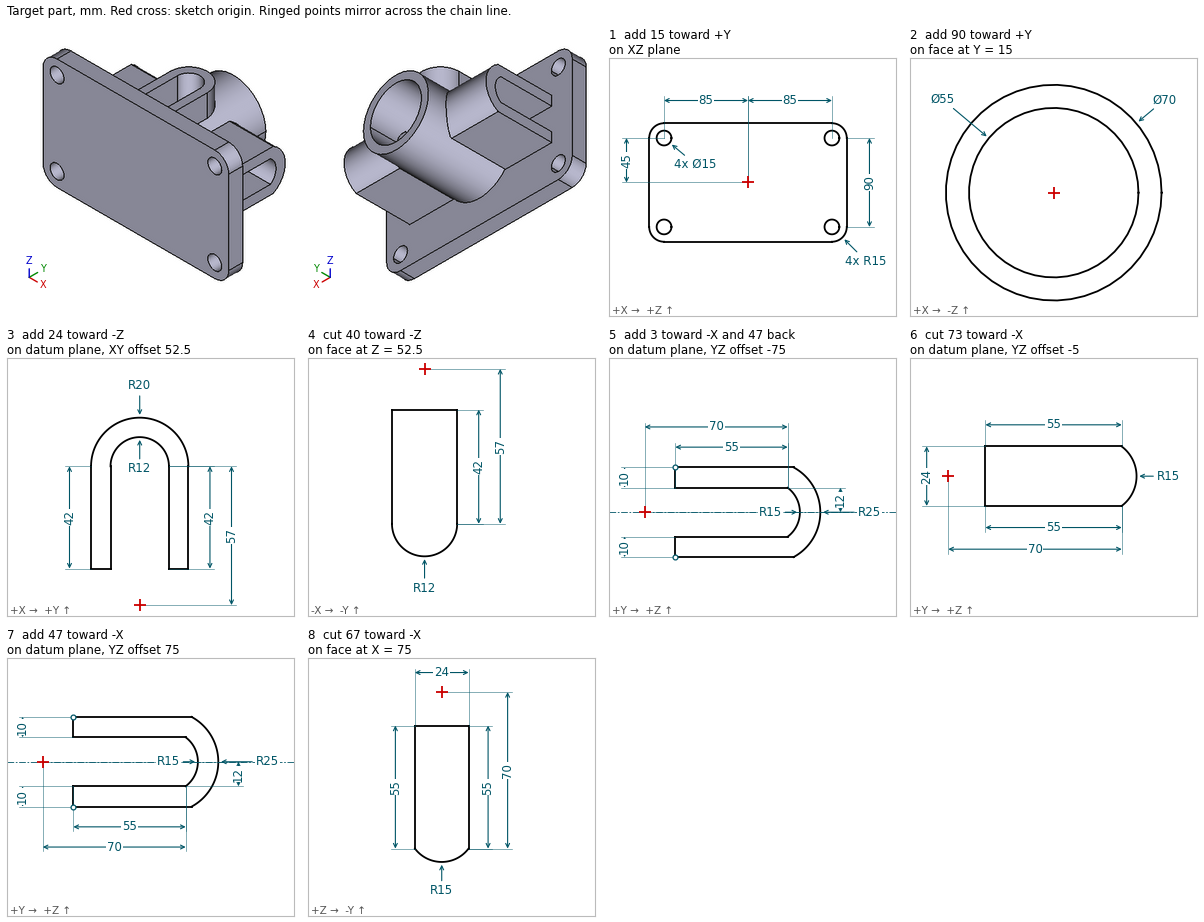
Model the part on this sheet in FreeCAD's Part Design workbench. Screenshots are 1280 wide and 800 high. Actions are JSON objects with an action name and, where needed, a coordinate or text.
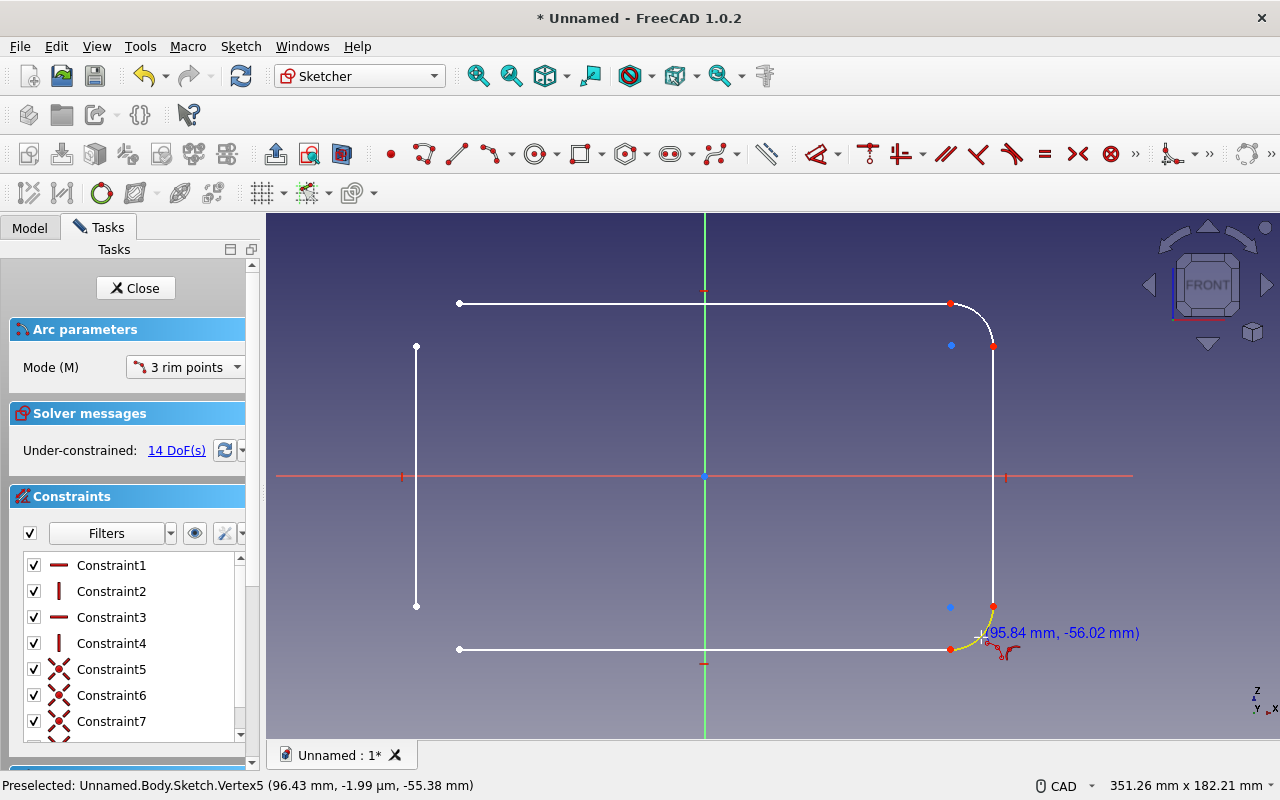
{"action": "left_click", "coordinate": [459, 650]}
{"action": "left_click", "coordinate": [416, 607]}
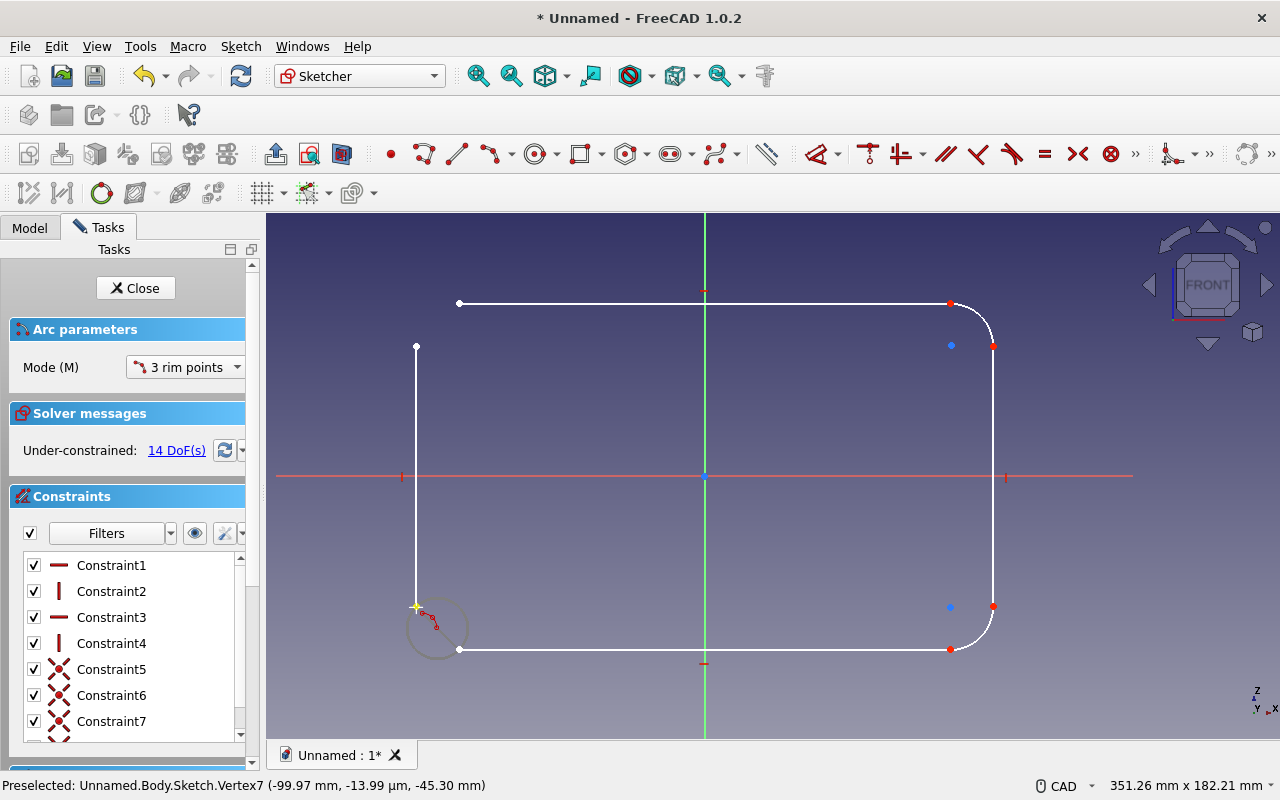
{"action": "scroll", "coordinate": [429, 637], "scroll_direction": "up", "scroll_amount": 2}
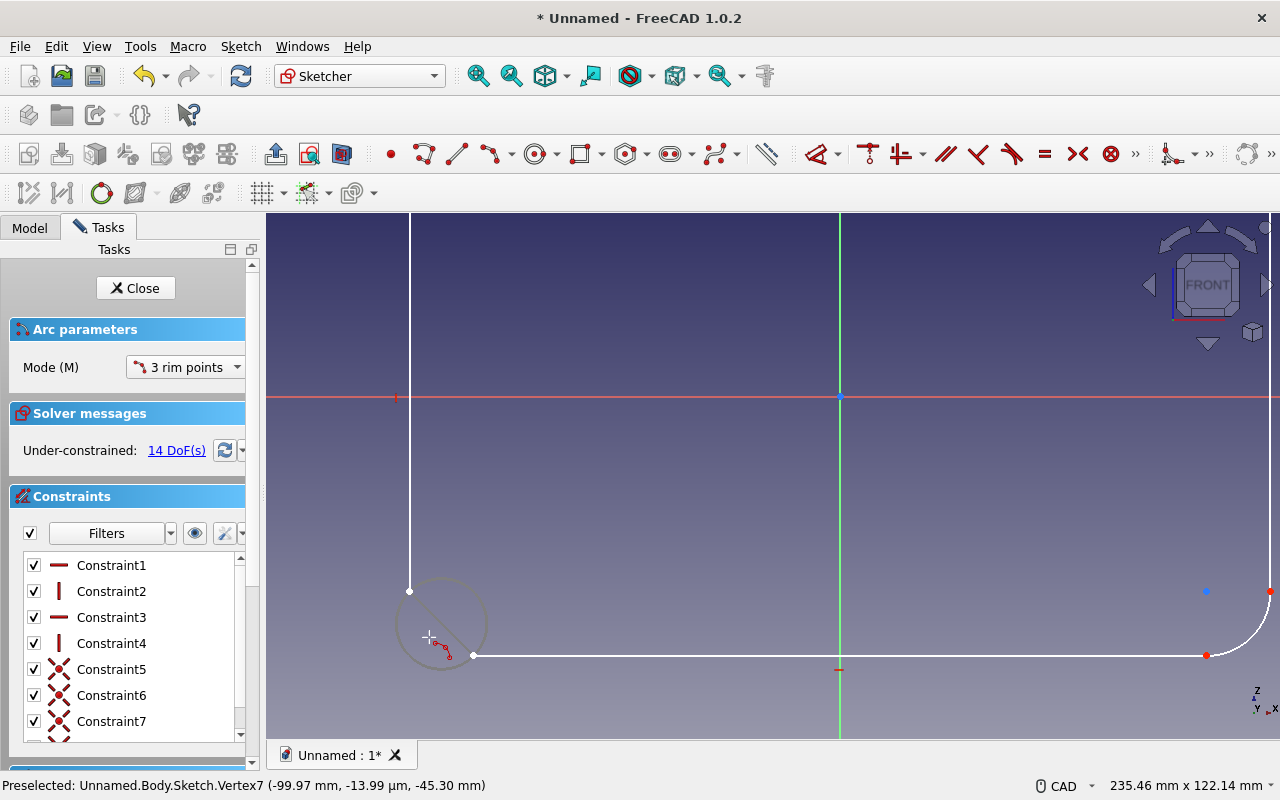
{"action": "left_click", "coordinate": [428, 636]}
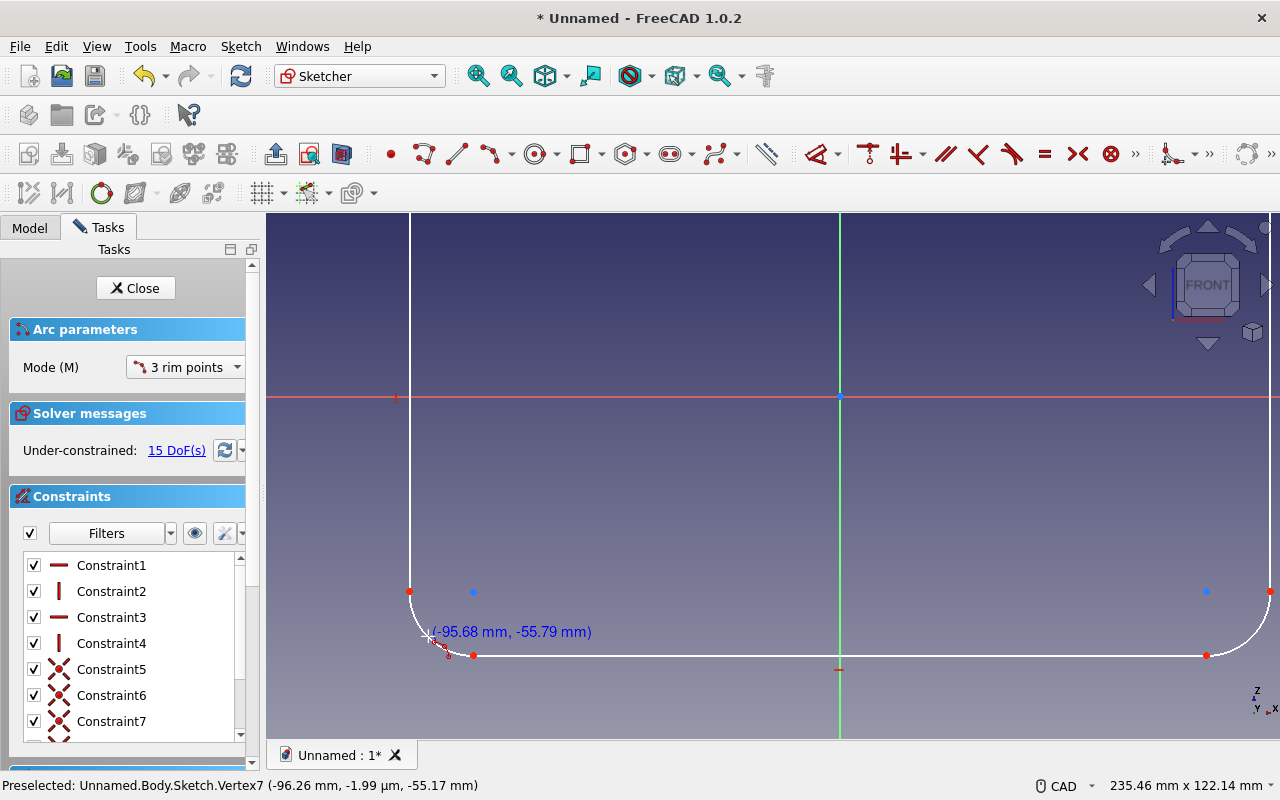
{"action": "scroll", "coordinate": [429, 637], "scroll_direction": "down", "scroll_amount": 2}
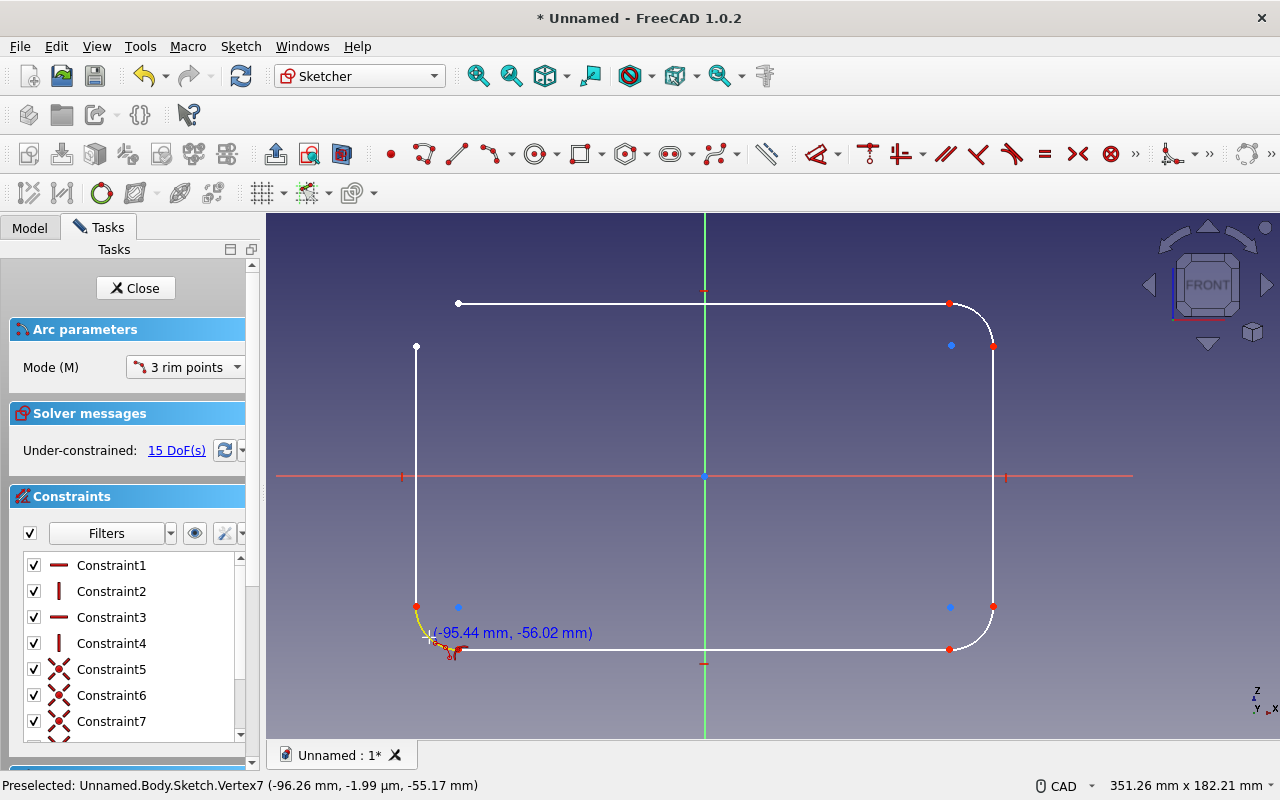
{"action": "left_click", "coordinate": [416, 347]}
{"action": "left_click", "coordinate": [459, 304]}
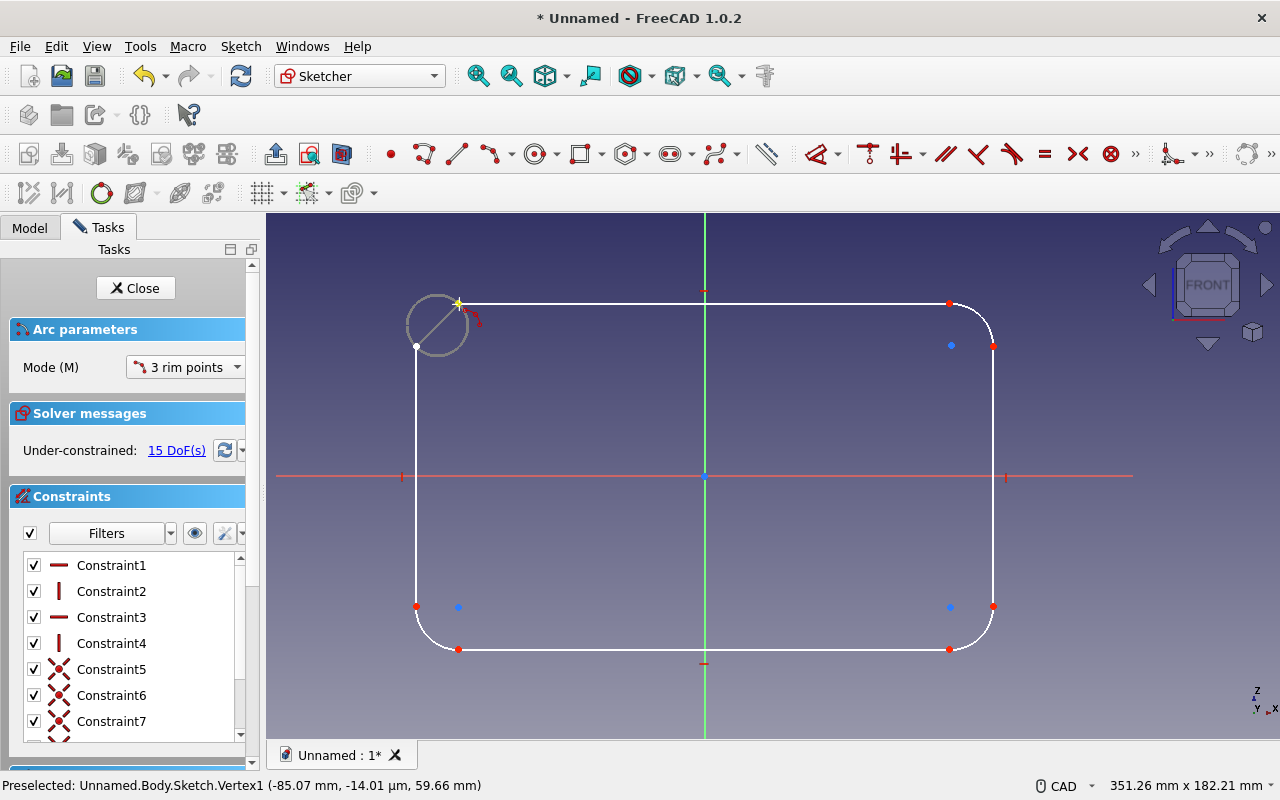
{"action": "scroll", "coordinate": [429, 316], "scroll_direction": "up", "scroll_amount": 2}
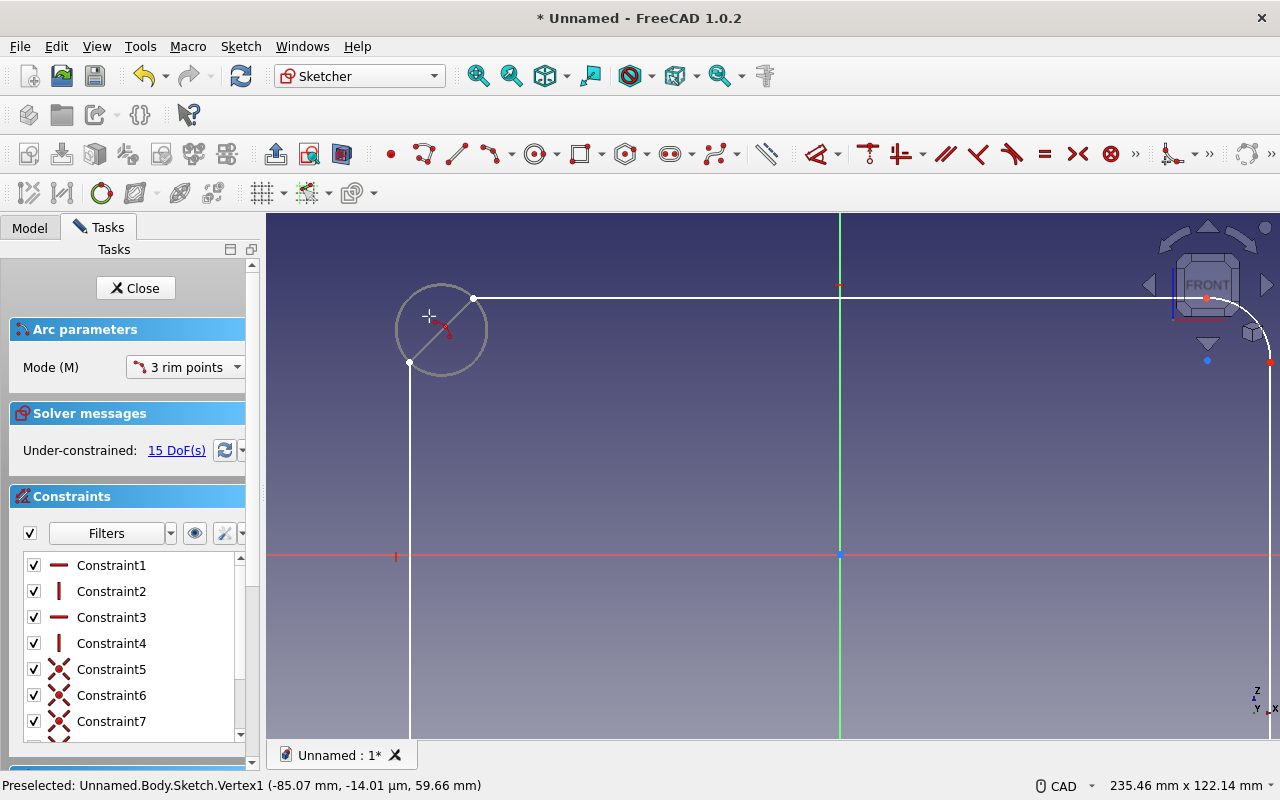
{"action": "left_click", "coordinate": [428, 315]}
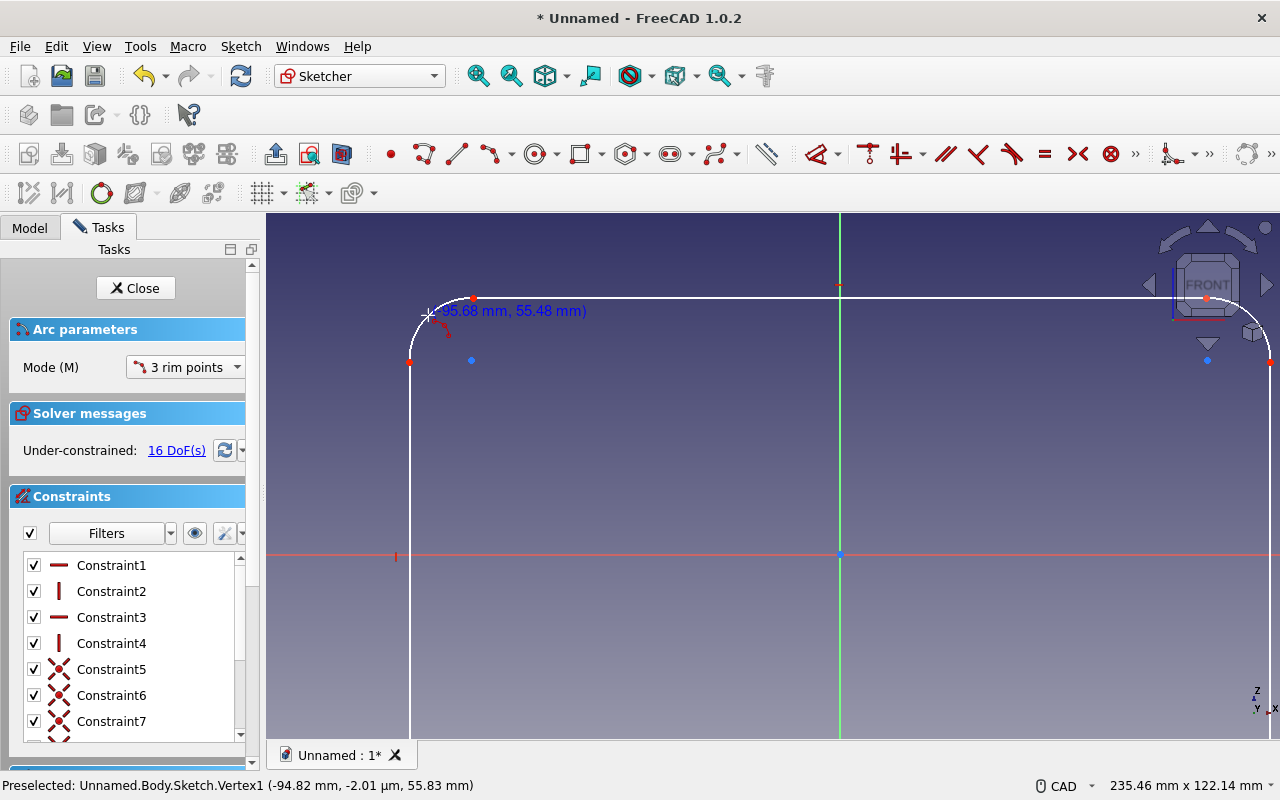
{"action": "key", "text": "g c"}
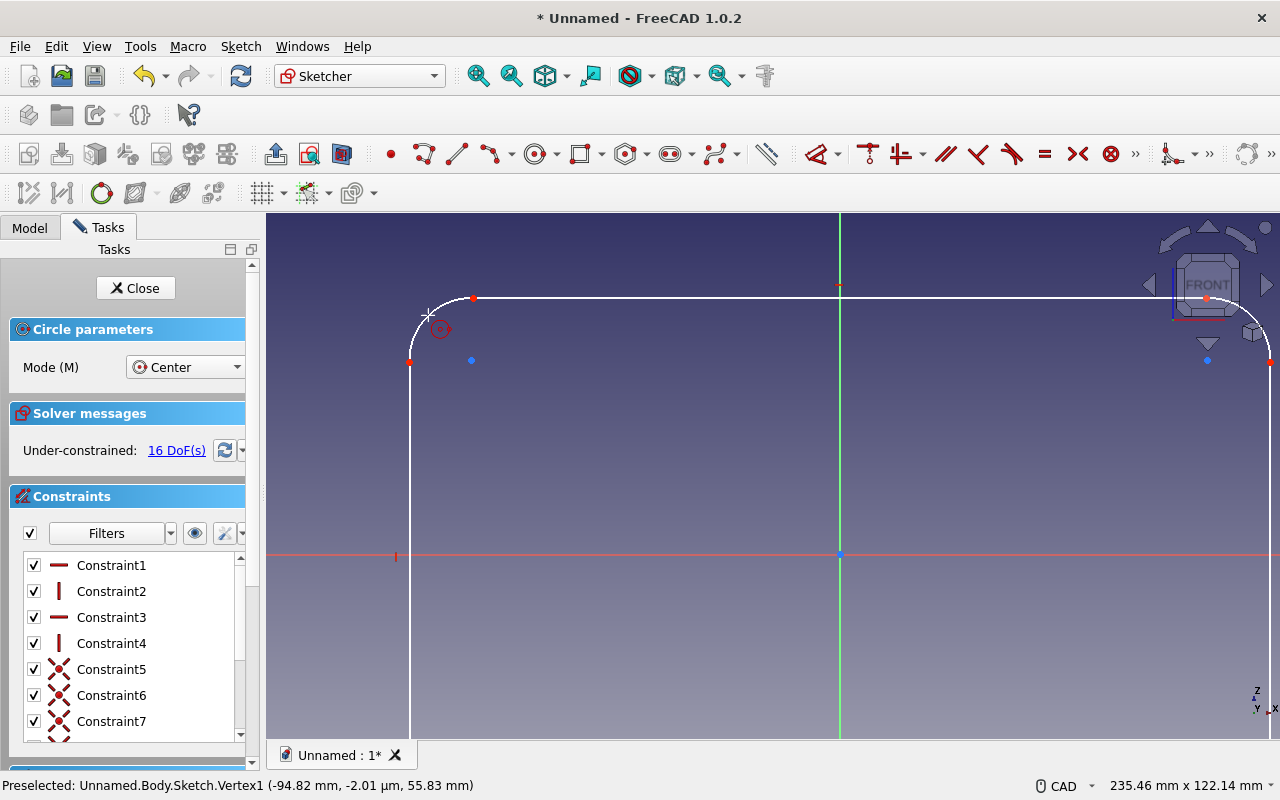
{"action": "left_click", "coordinate": [474, 361]}
{"action": "mouse_move", "coordinate": [497, 338]}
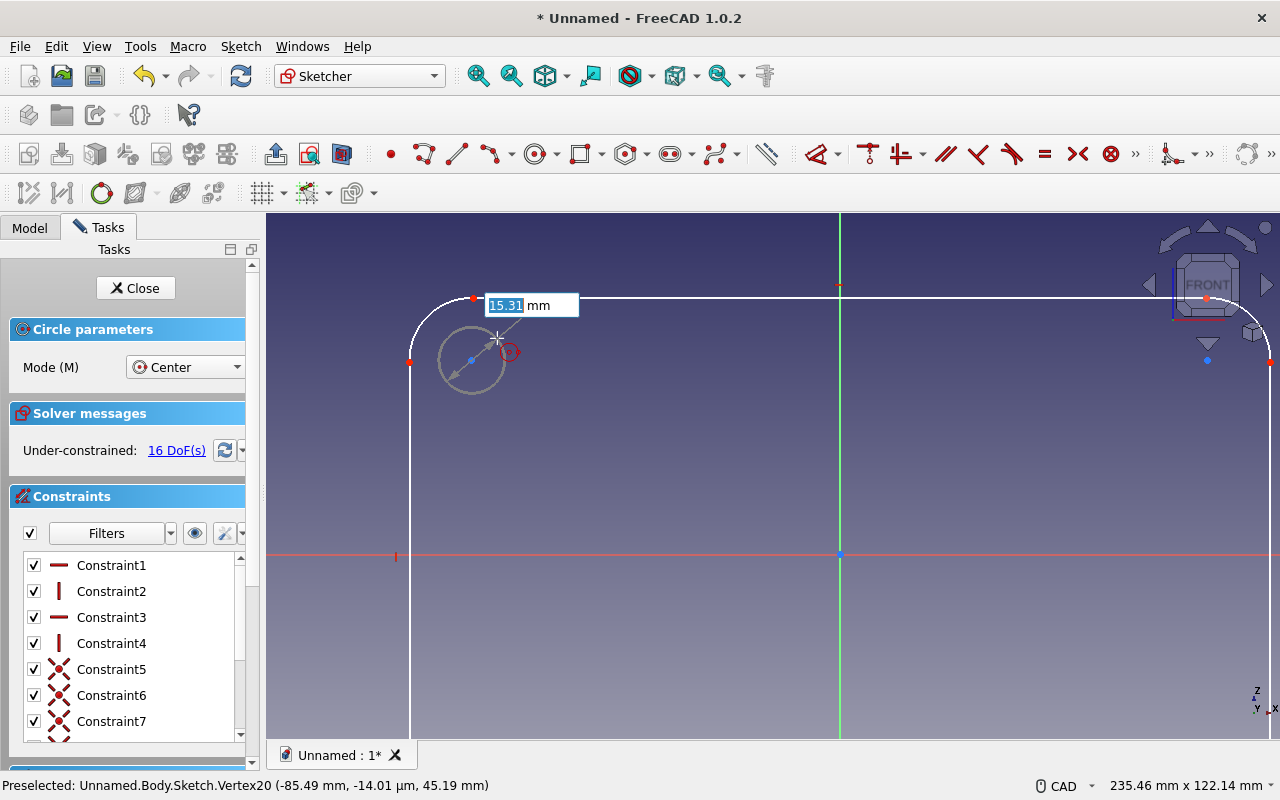
{"action": "type", "text": "15"}
{"action": "key", "text": "Return"}